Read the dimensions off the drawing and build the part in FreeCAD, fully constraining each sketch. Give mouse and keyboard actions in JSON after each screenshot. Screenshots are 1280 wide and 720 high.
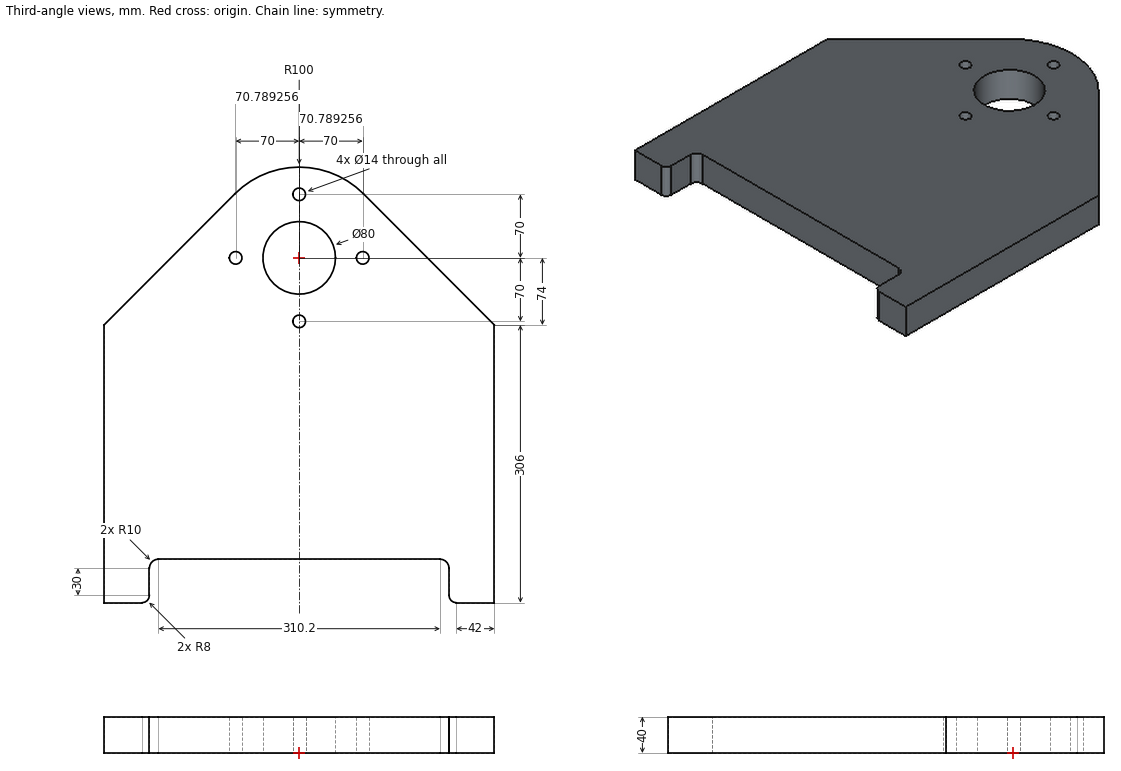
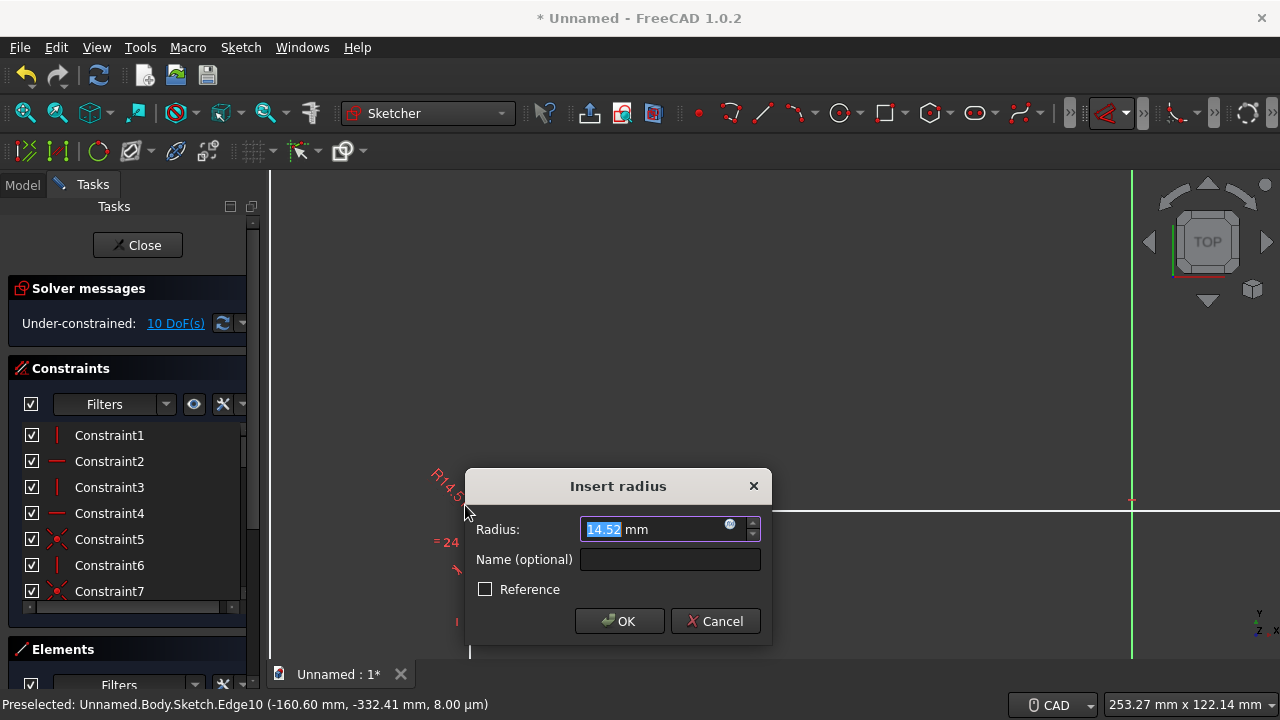
{"action": "type", "text": "10"}
{"action": "key", "text": "Return"}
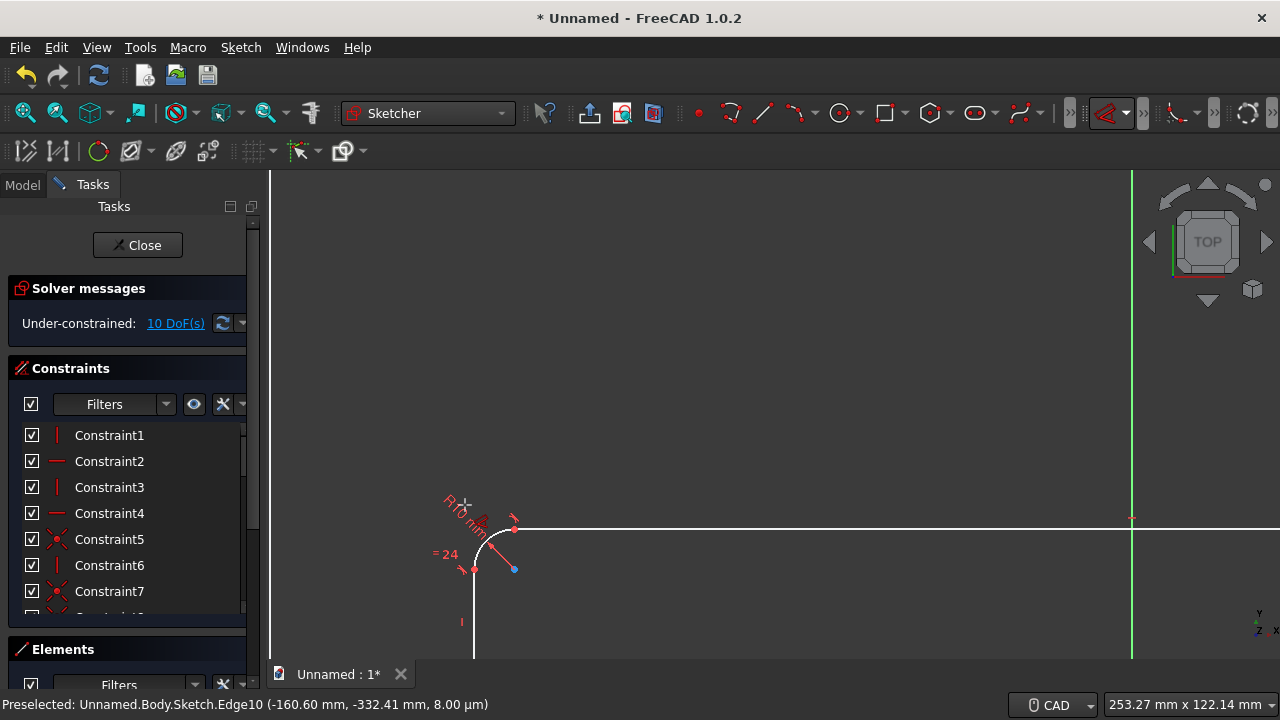
{"action": "scroll", "coordinate": [620, 545], "scroll_direction": "down", "scroll_amount": 9}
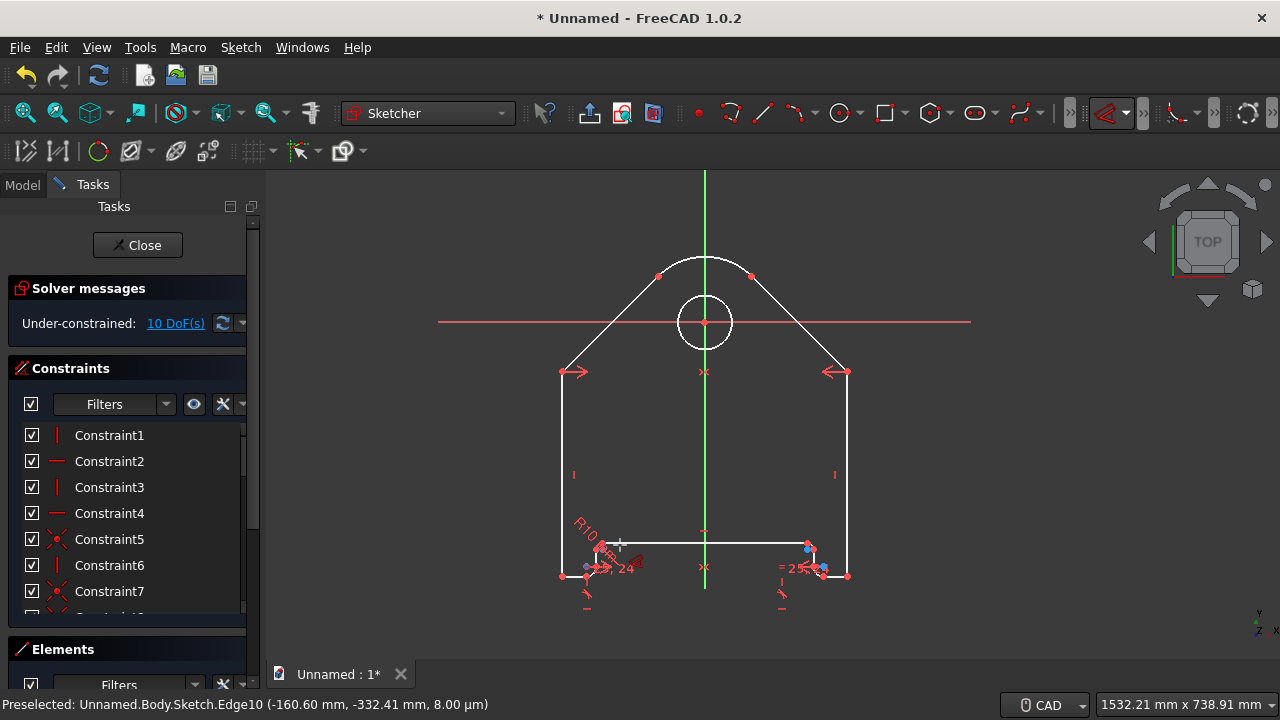
{"action": "scroll", "coordinate": [815, 571], "scroll_direction": "up", "scroll_amount": 11}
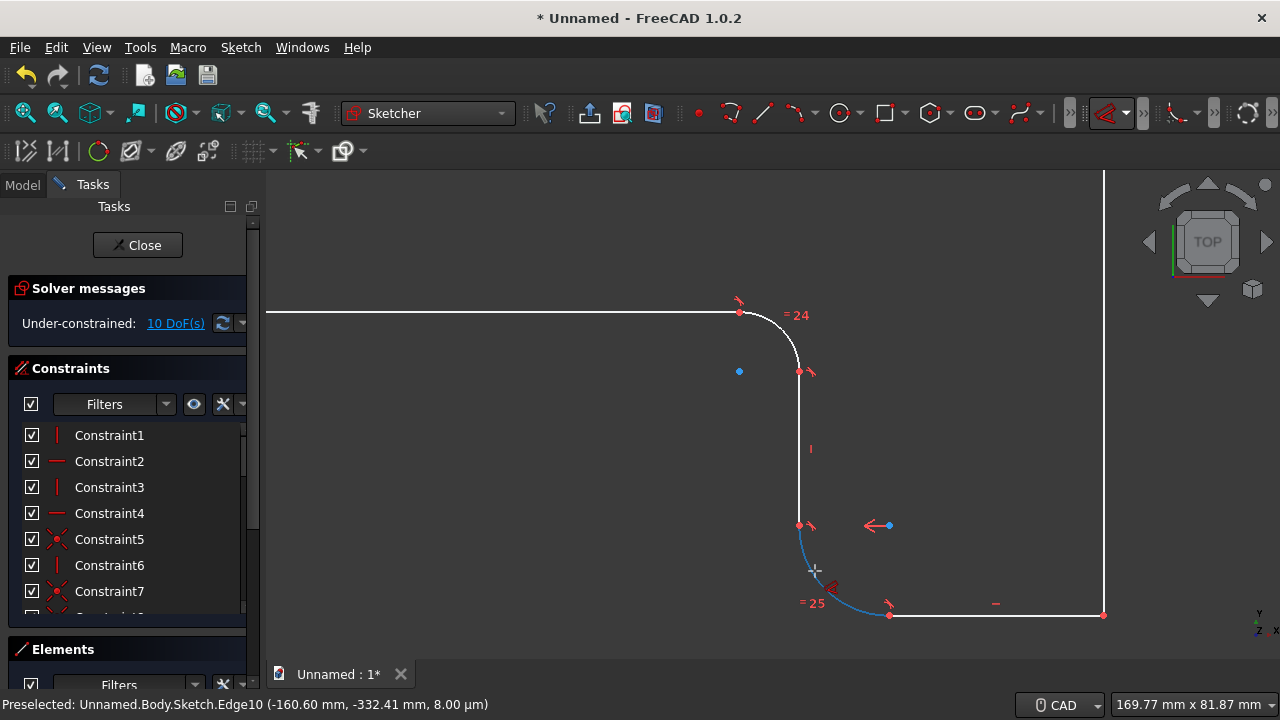
{"action": "left_click", "coordinate": [809, 567]}
{"action": "left_click", "coordinate": [781, 582]}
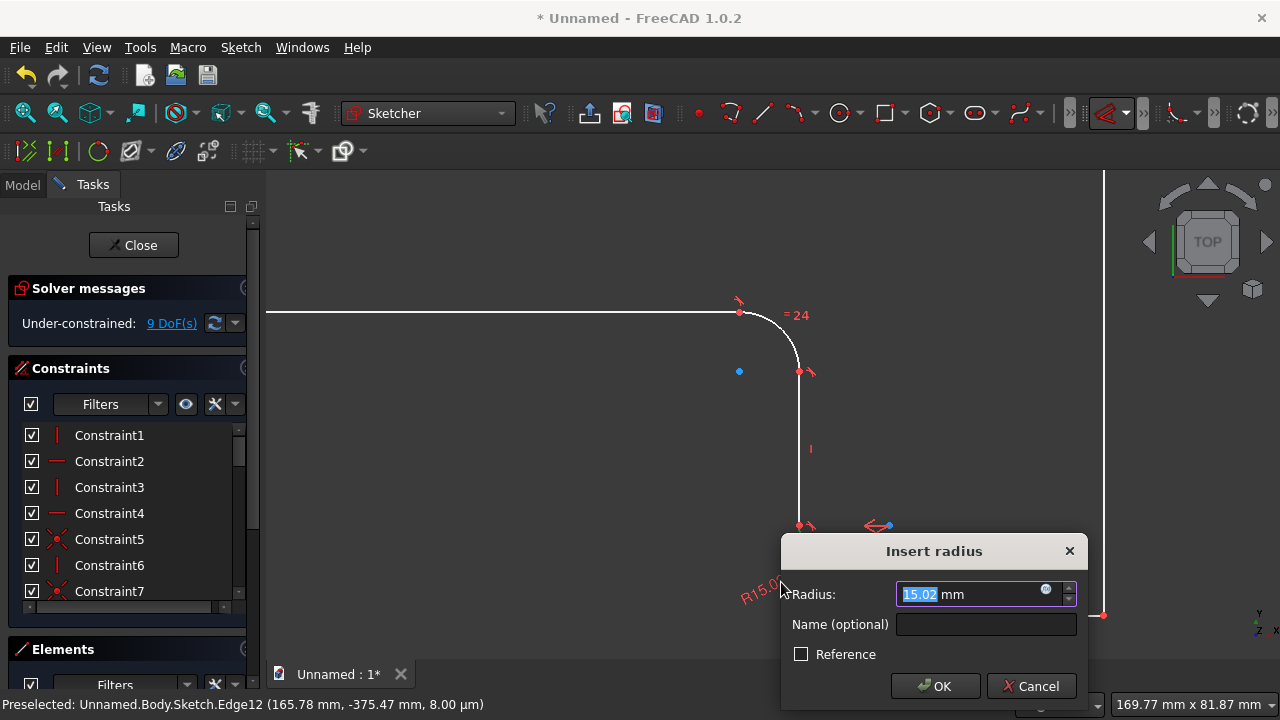
{"action": "type", "text": "8"}
{"action": "key", "text": "Return"}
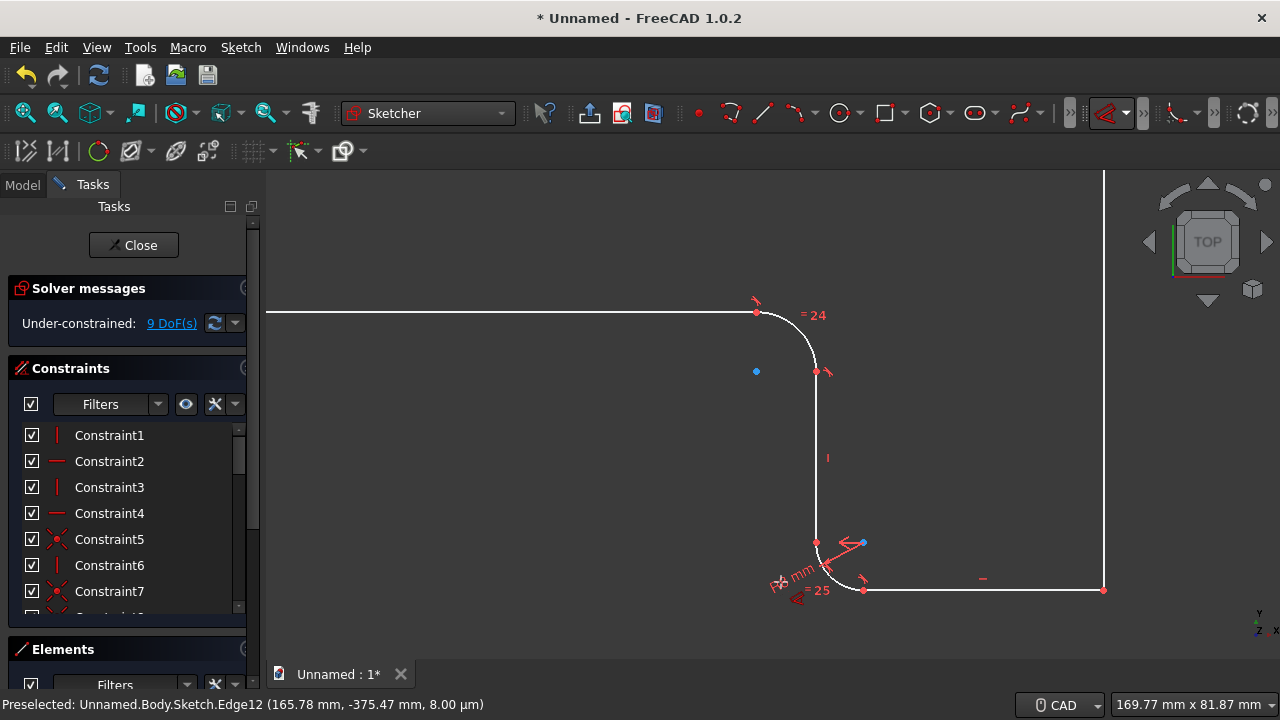
{"action": "scroll", "coordinate": [815, 571], "scroll_direction": "down", "scroll_amount": 11}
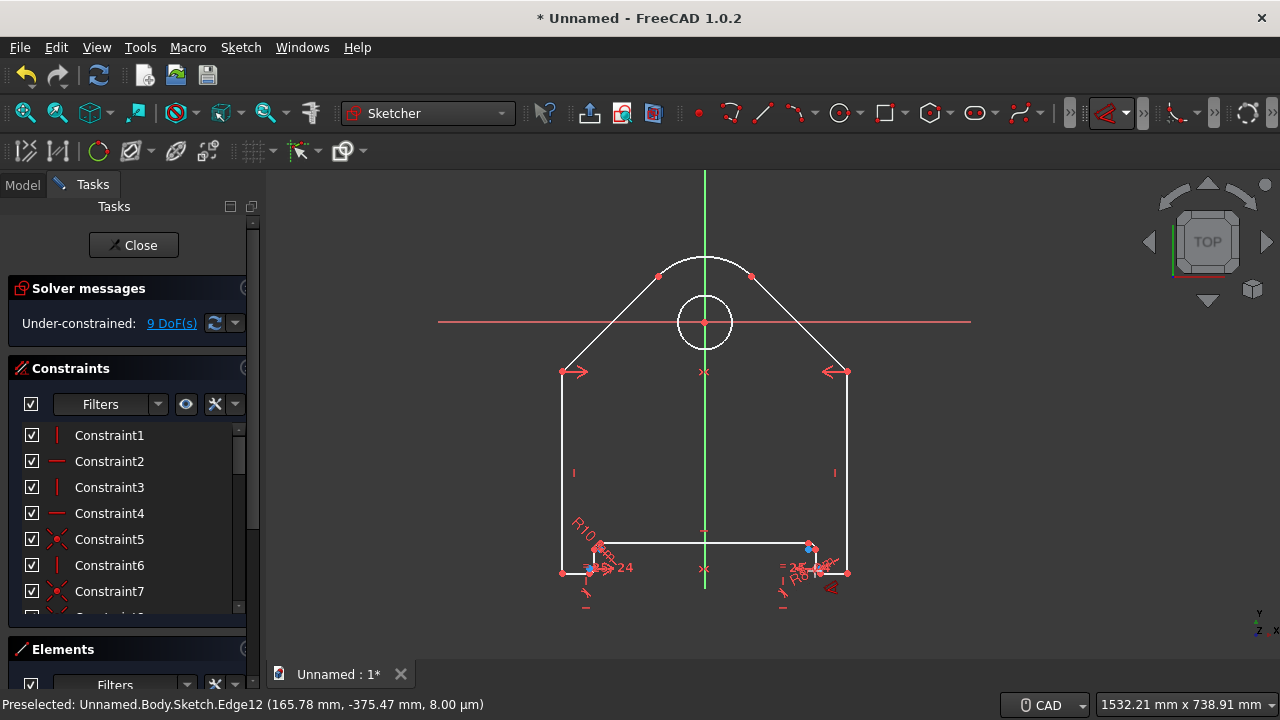
{"action": "left_click", "coordinate": [725, 260]}
{"action": "left_click", "coordinate": [735, 230]}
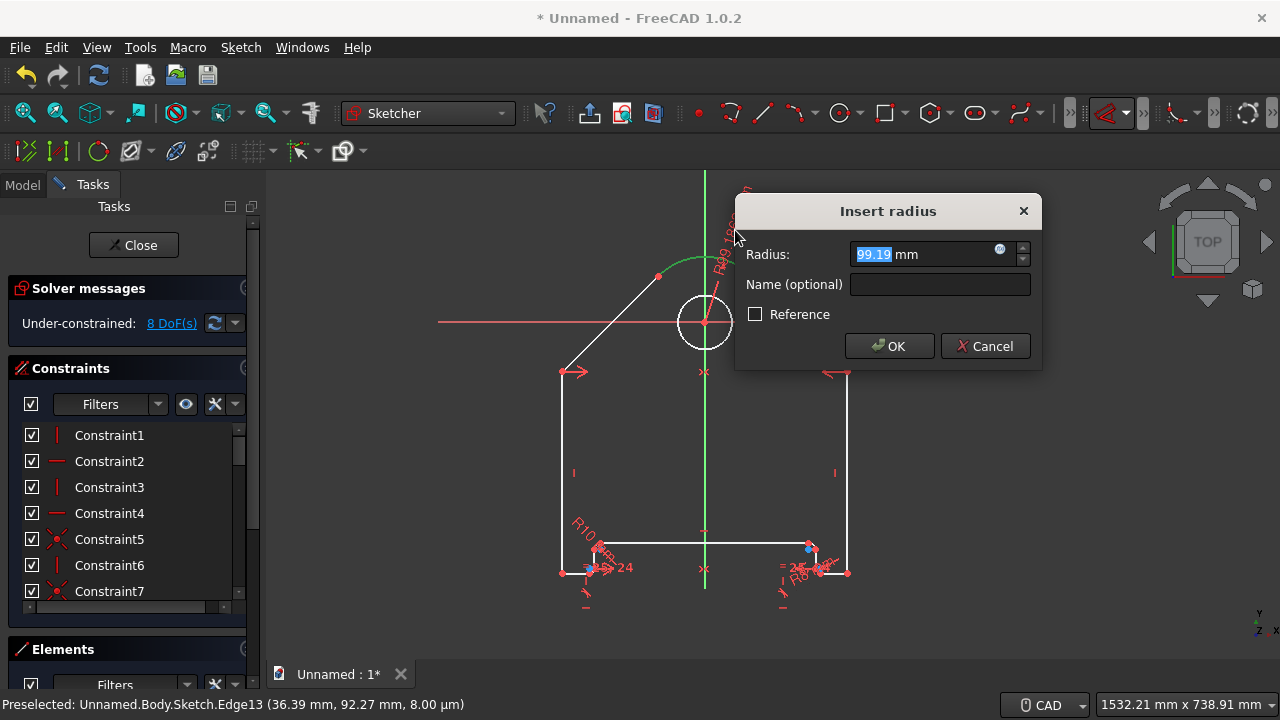
{"action": "type", "text": "100"}
{"action": "key", "text": "Return"}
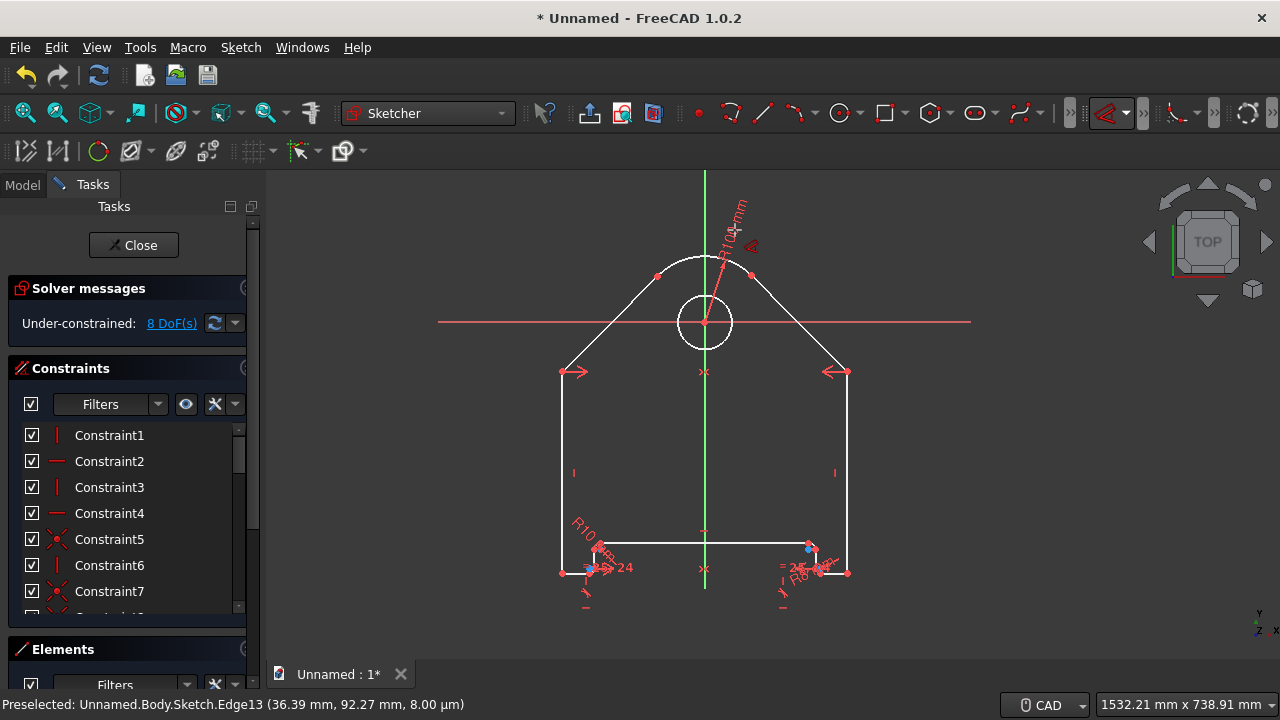
{"action": "left_click", "coordinate": [724, 303]}
{"action": "left_click", "coordinate": [762, 305]}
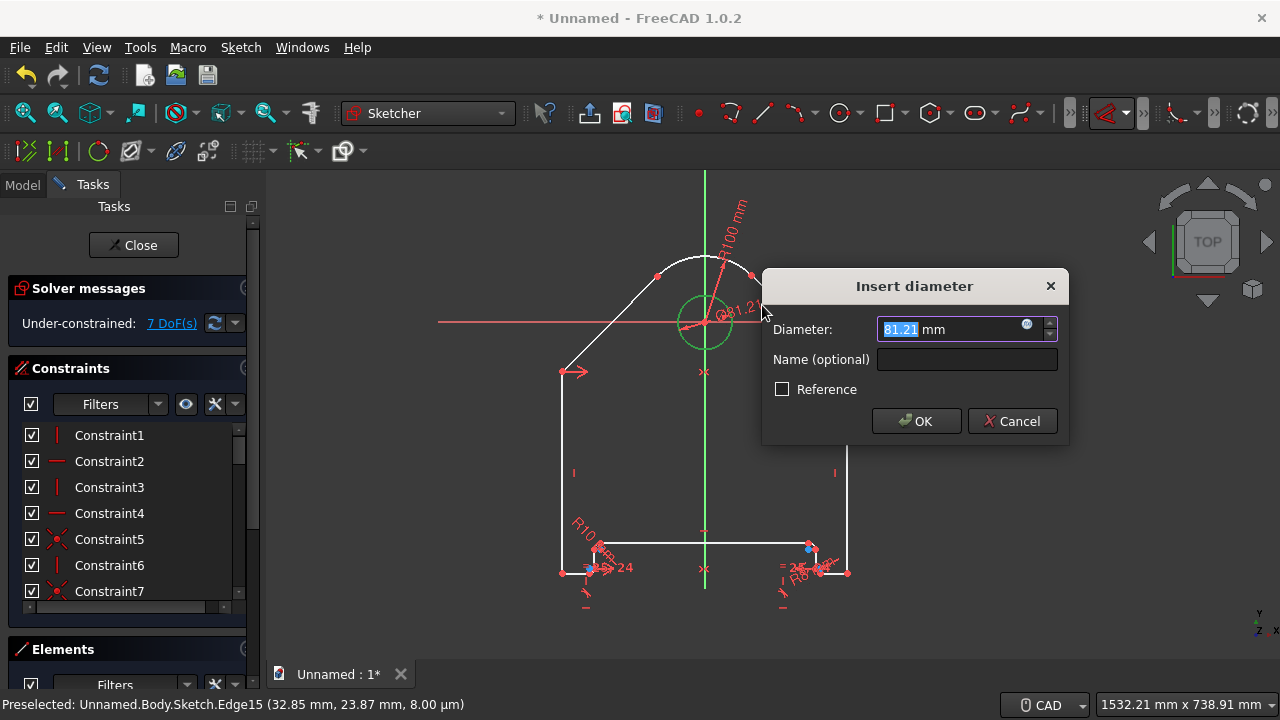
{"action": "type", "text": "80"}
{"action": "key", "text": "Return"}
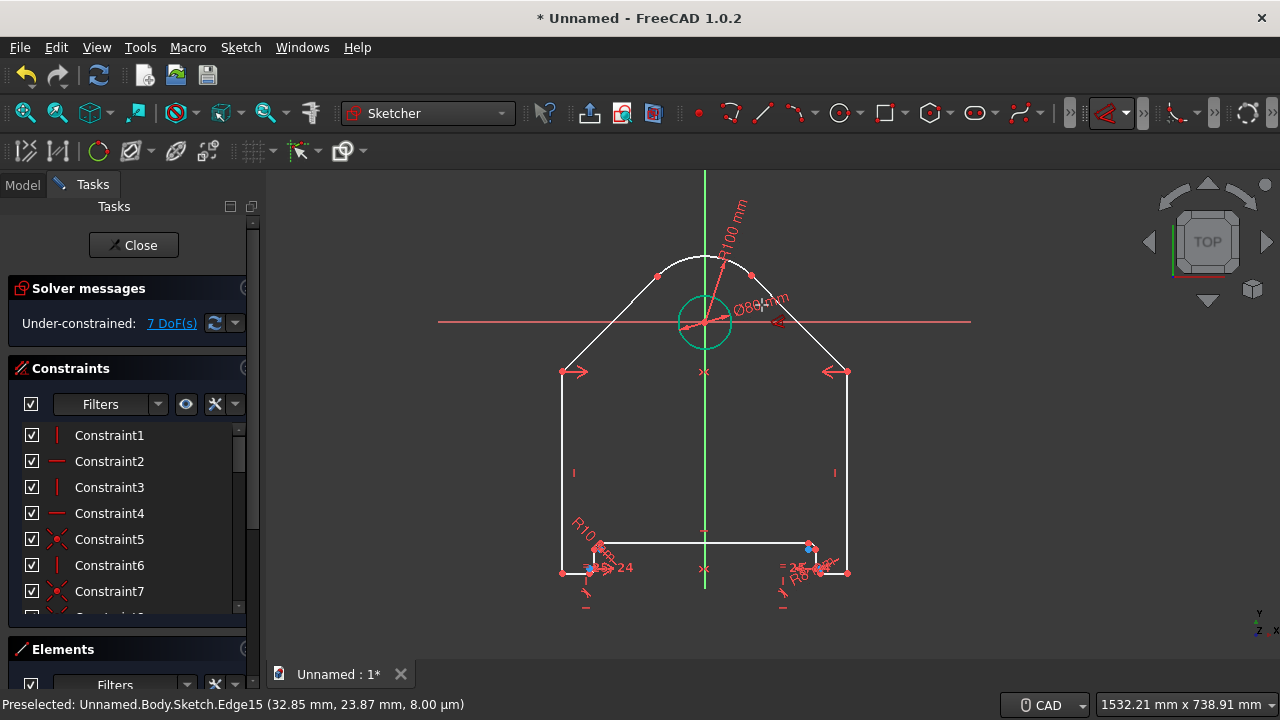
{"action": "scroll", "coordinate": [594, 559], "scroll_direction": "up", "scroll_amount": 4}